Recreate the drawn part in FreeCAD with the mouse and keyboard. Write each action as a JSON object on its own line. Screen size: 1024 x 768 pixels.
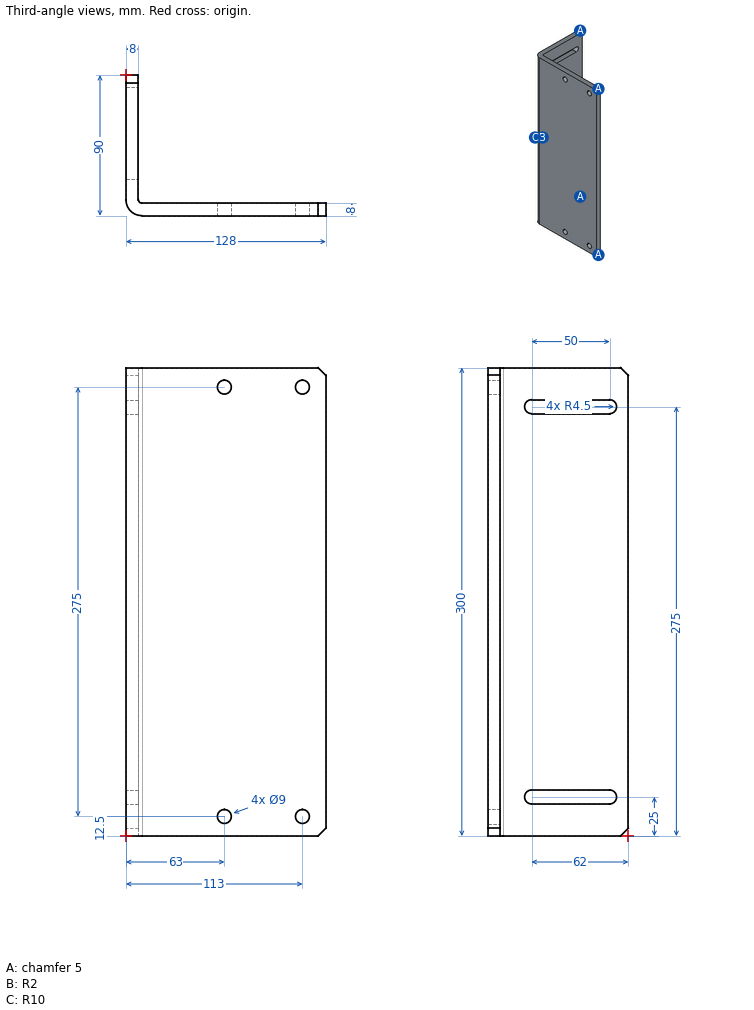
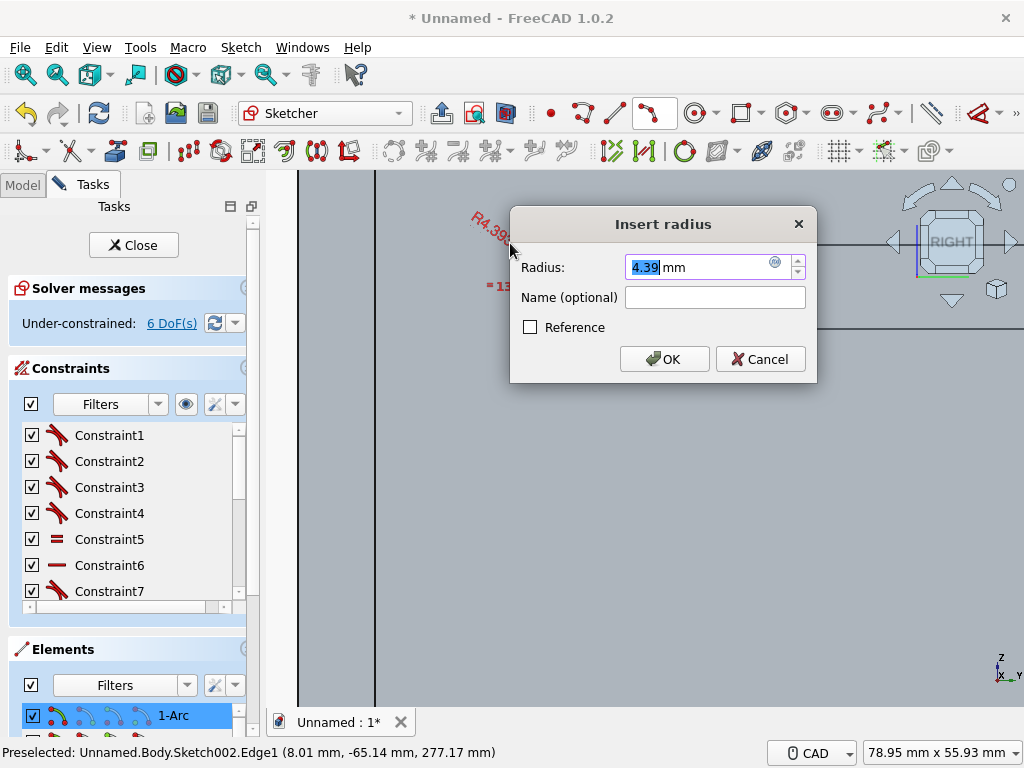
{"action": "type", "text": "4.5"}
{"action": "key", "text": "Return"}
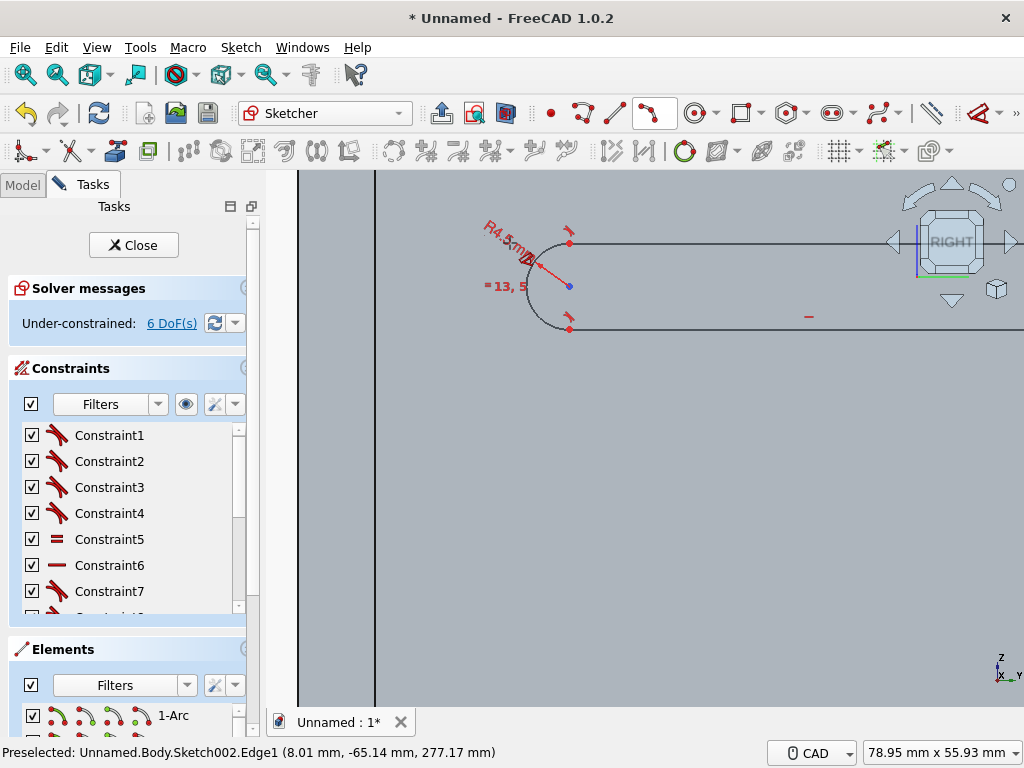
{"action": "scroll", "coordinate": [535, 260], "scroll_direction": "down", "scroll_amount": 10}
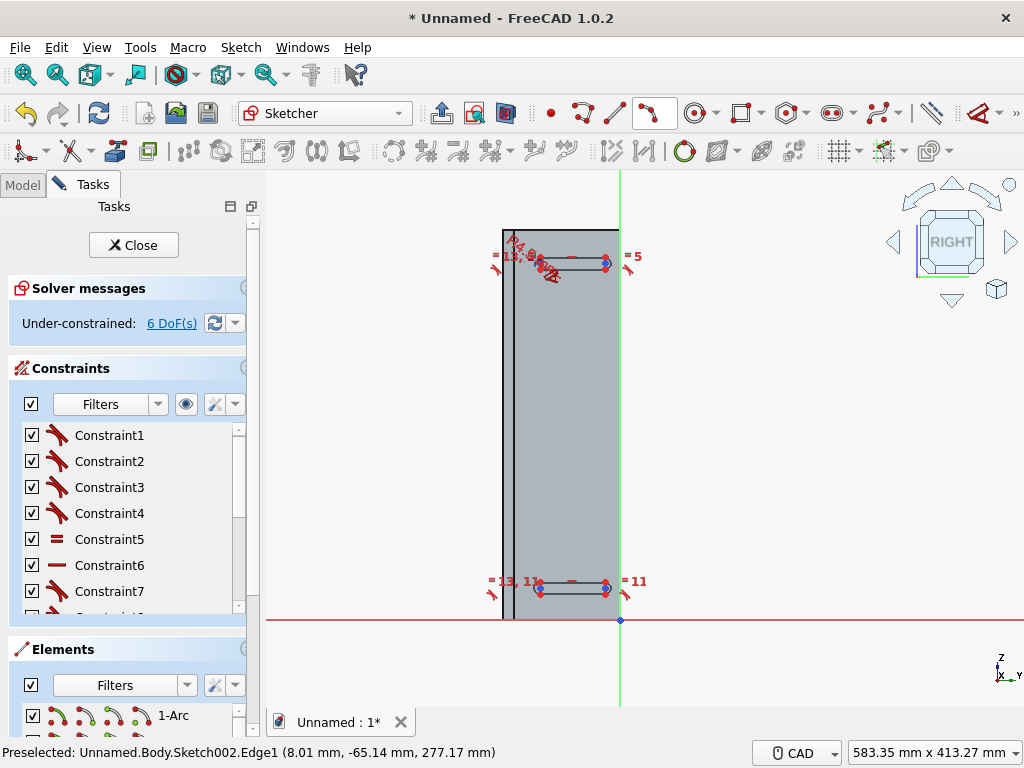
{"action": "left_click", "coordinate": [559, 258]}
{"action": "left_click", "coordinate": [572, 224]}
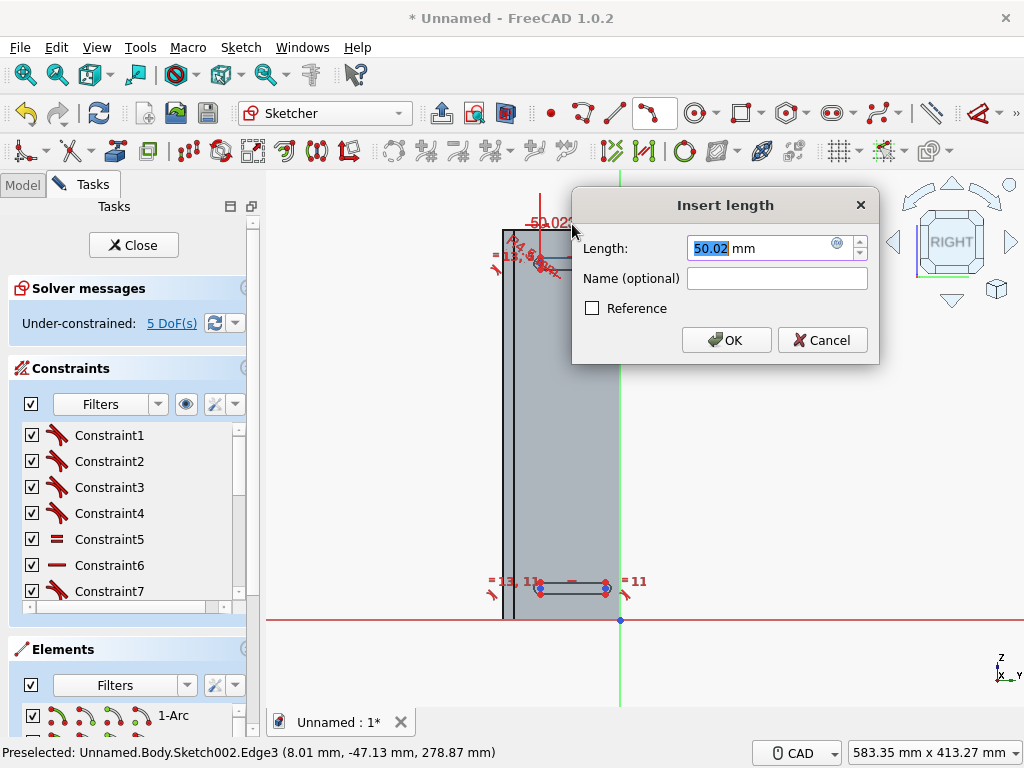
{"action": "type", "text": "50"}
{"action": "key", "text": "Return"}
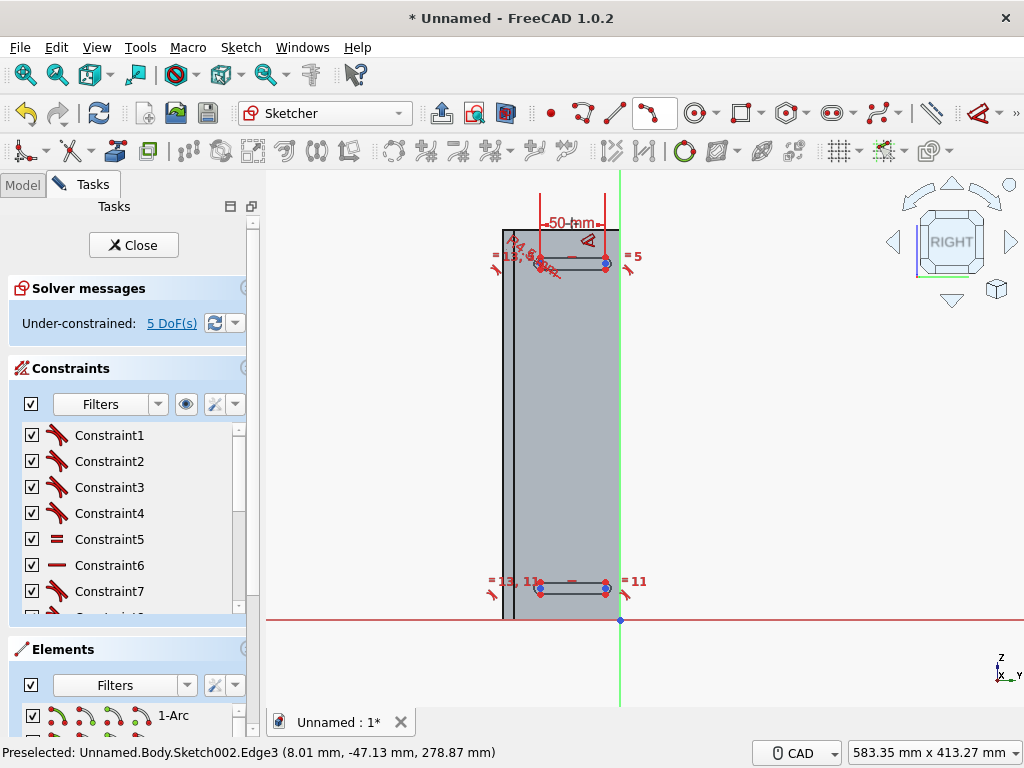
{"action": "left_click", "coordinate": [559, 583]}
{"action": "left_click", "coordinate": [572, 549]}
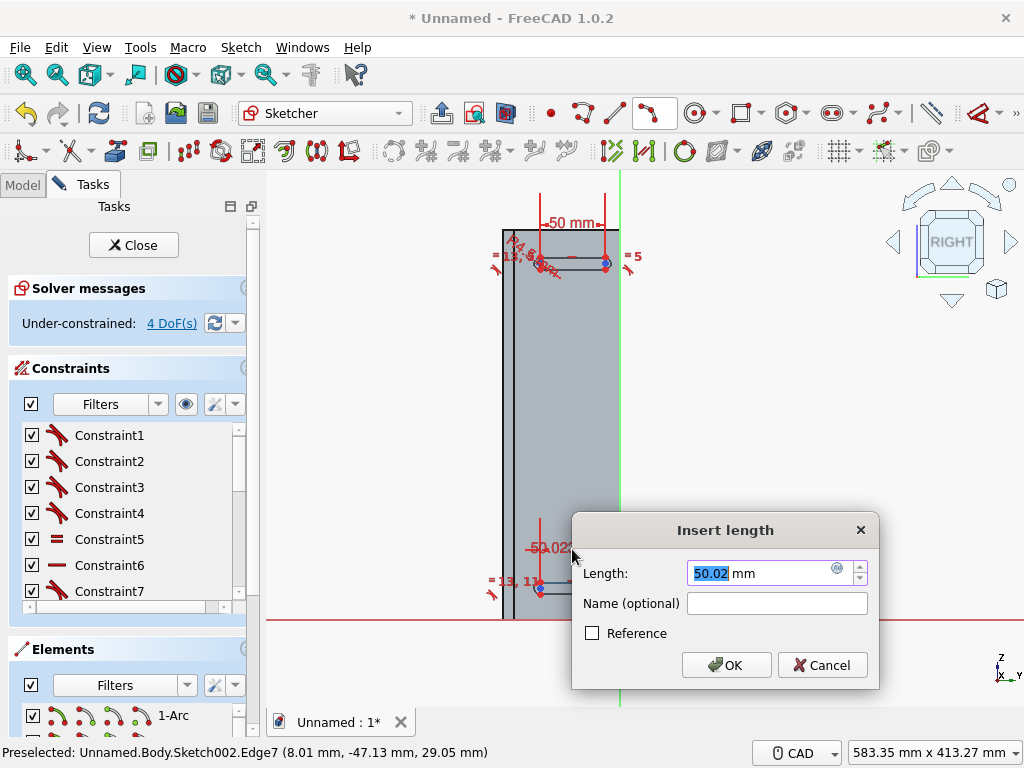
{"action": "type", "text": "50"}
{"action": "key", "text": "Return"}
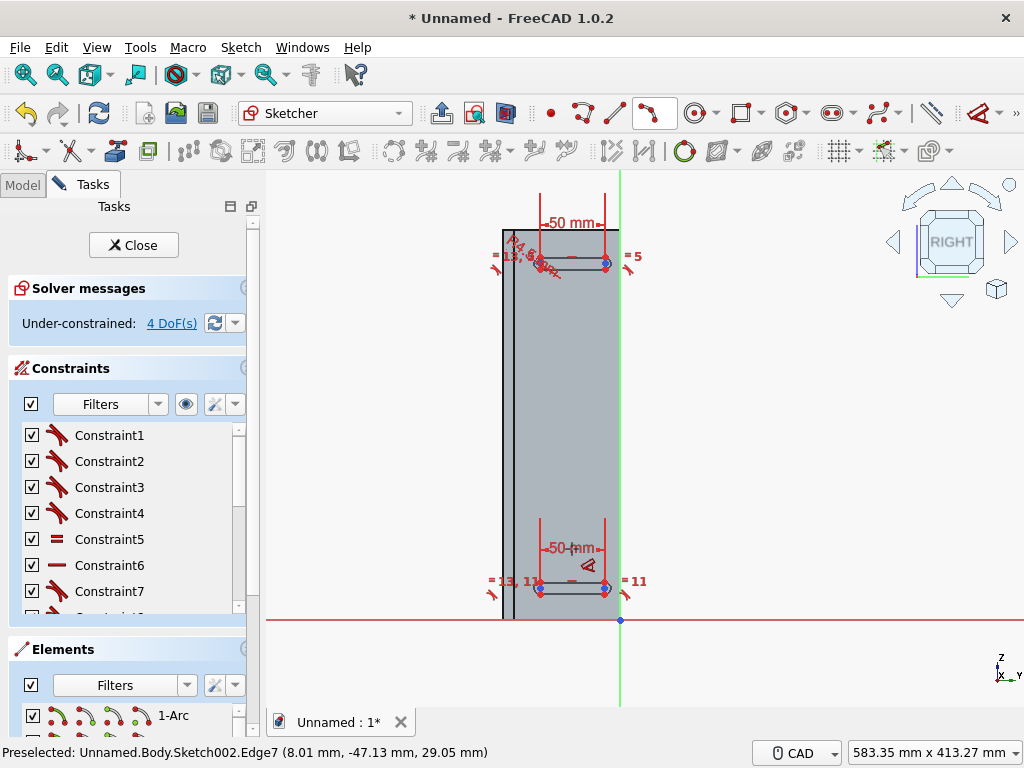
{"action": "scroll", "coordinate": [540, 258], "scroll_direction": "up", "scroll_amount": 4}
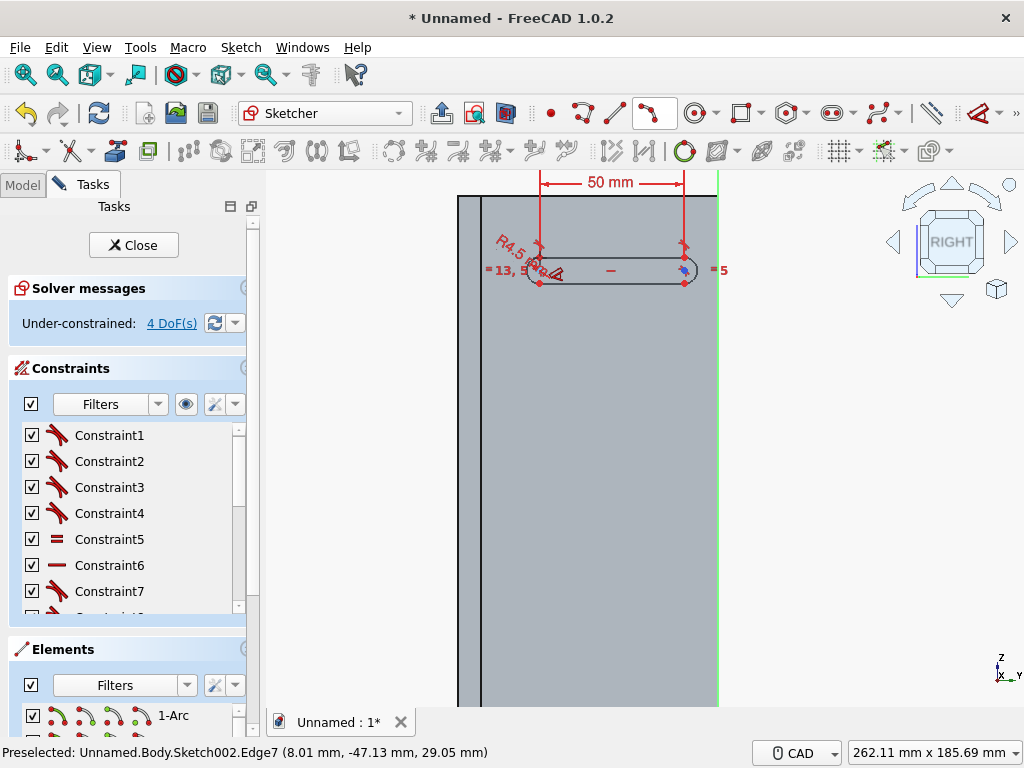
{"action": "left_click", "coordinate": [540, 258]}
{"action": "left_click", "coordinate": [629, 224]}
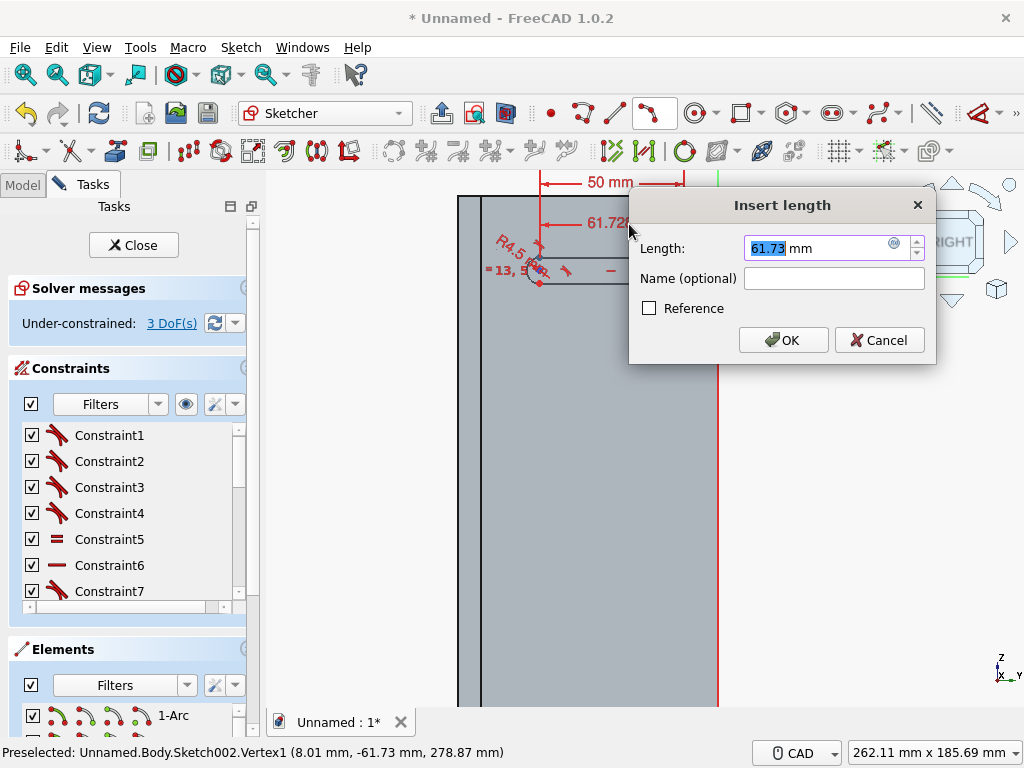
{"action": "type", "text": "62"}
{"action": "key", "text": "Return"}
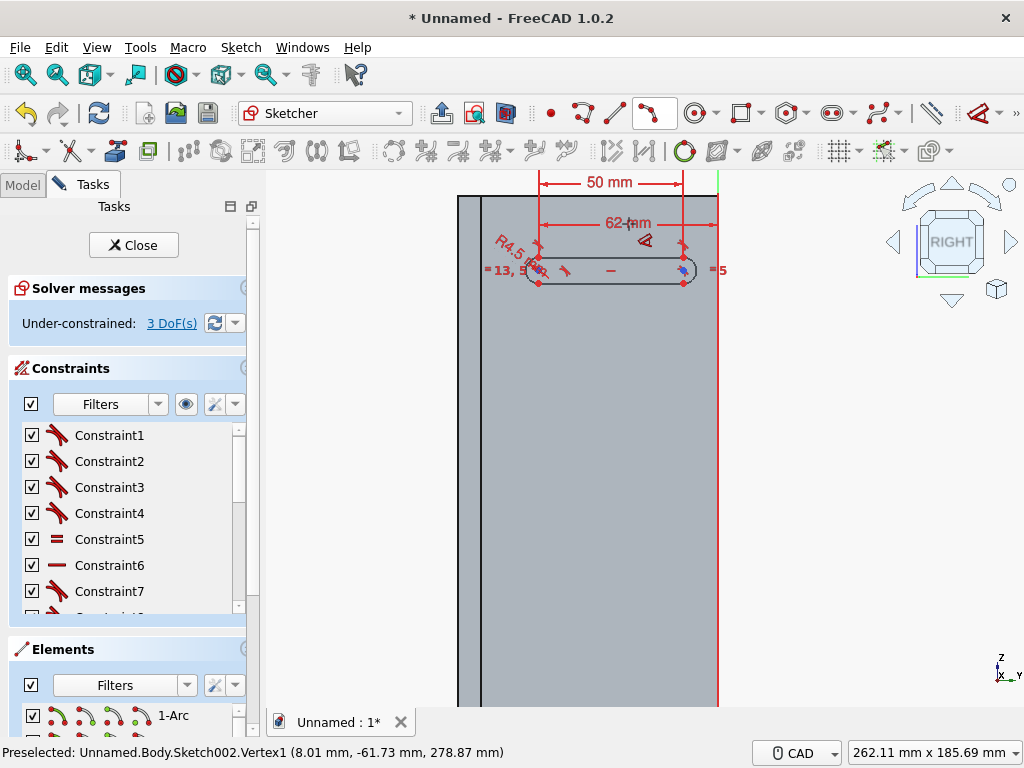
{"action": "scroll", "coordinate": [539, 258], "scroll_direction": "down", "scroll_amount": 4}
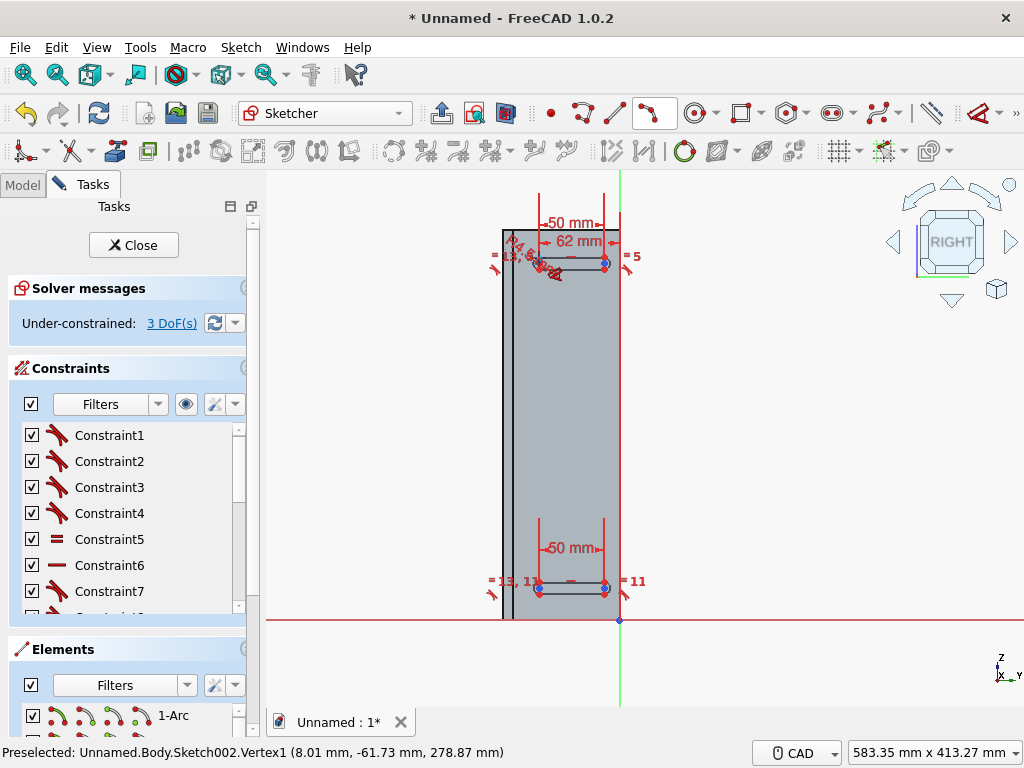
{"action": "scroll", "coordinate": [539, 583], "scroll_direction": "up", "scroll_amount": 4}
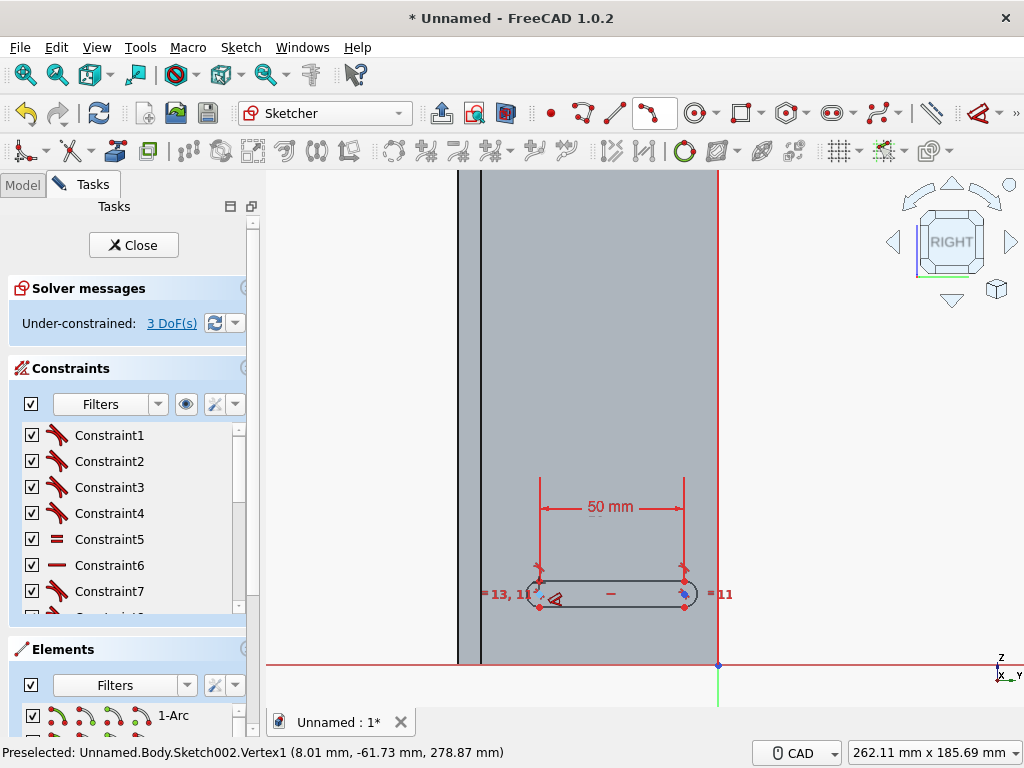
{"action": "left_click", "coordinate": [540, 581]}
{"action": "left_click", "coordinate": [629, 547]}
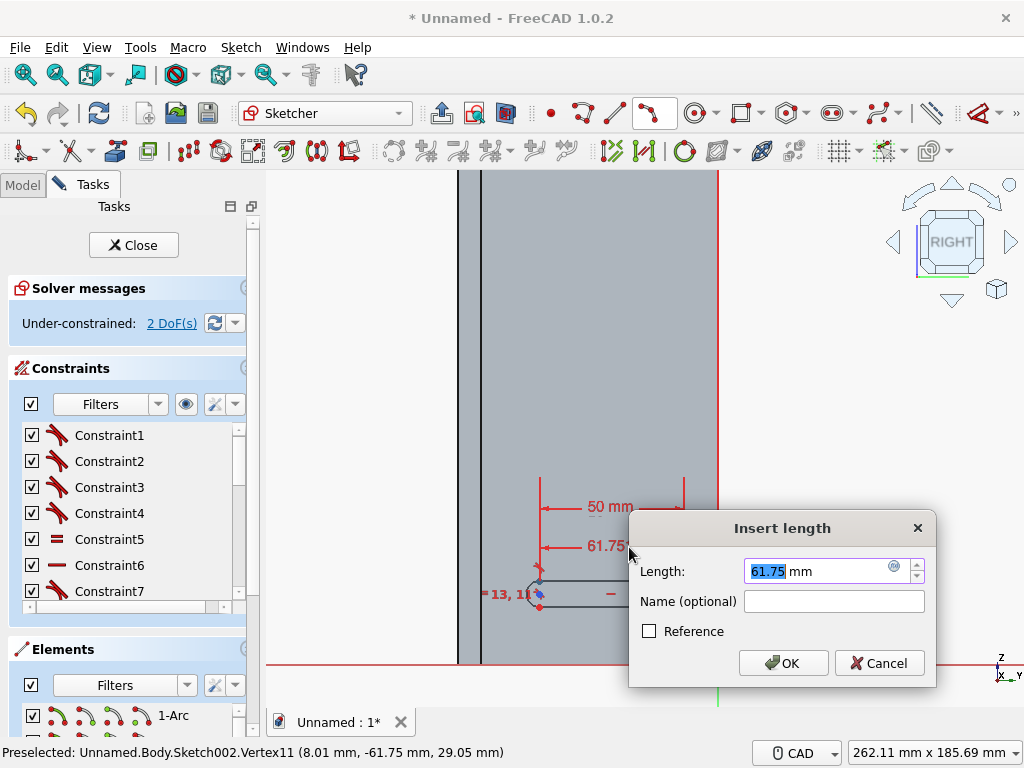
{"action": "type", "text": "62"}
{"action": "key", "text": "Return"}